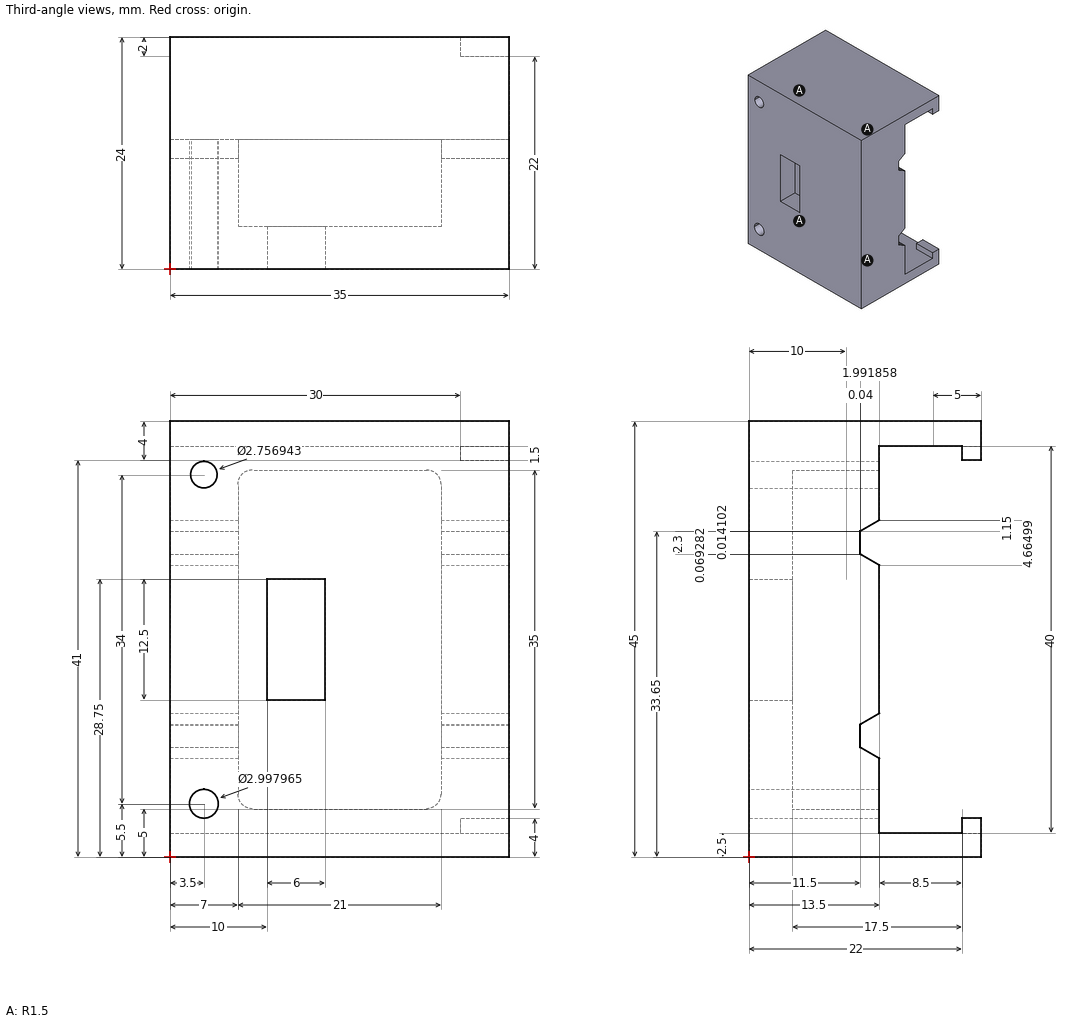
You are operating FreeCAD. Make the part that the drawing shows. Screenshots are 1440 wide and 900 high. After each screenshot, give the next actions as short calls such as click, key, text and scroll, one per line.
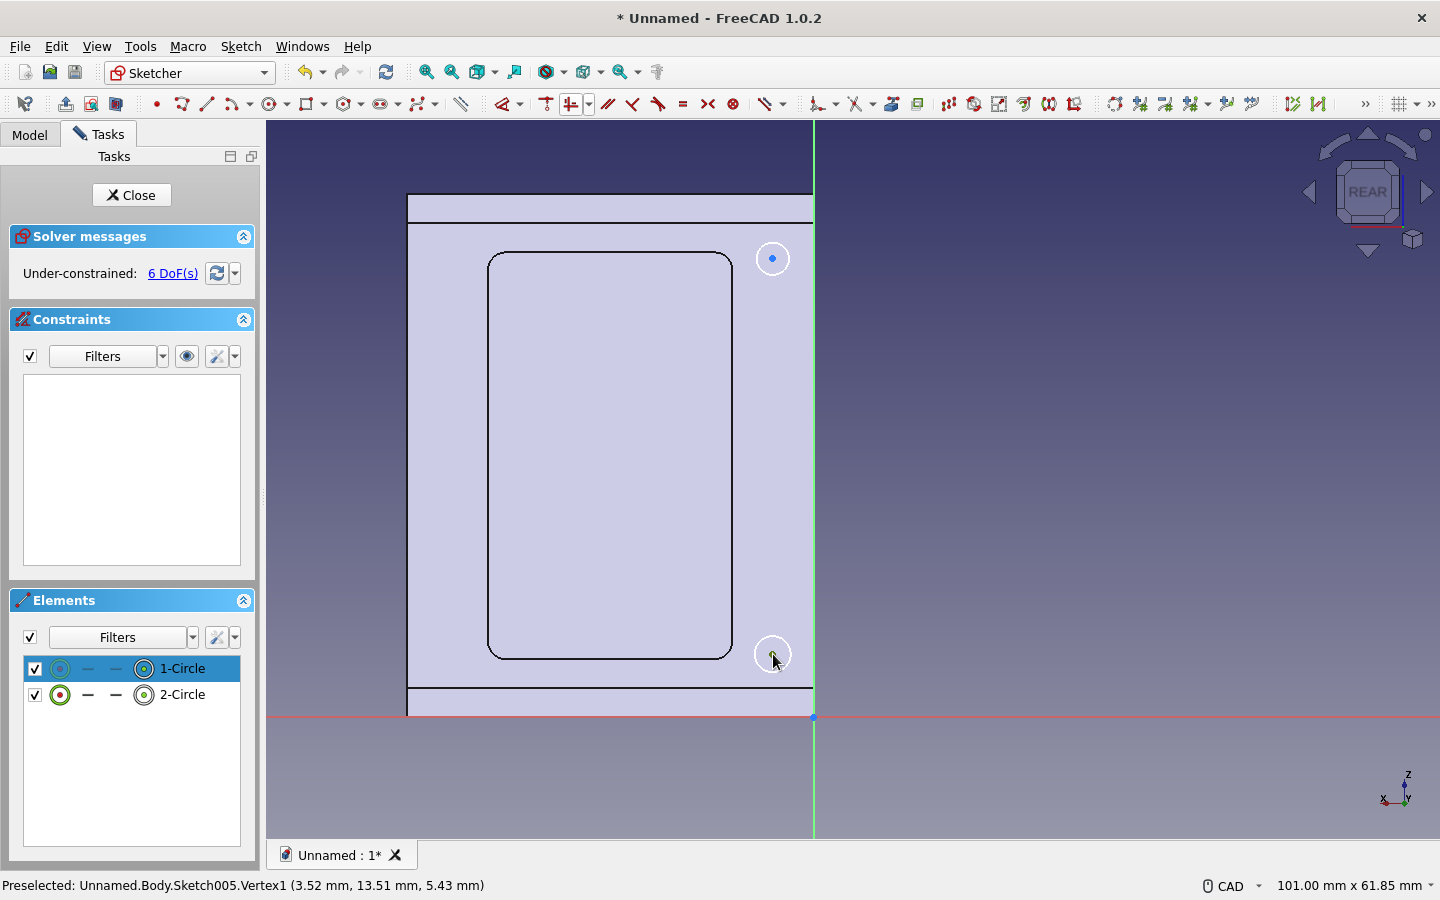
click(773, 259)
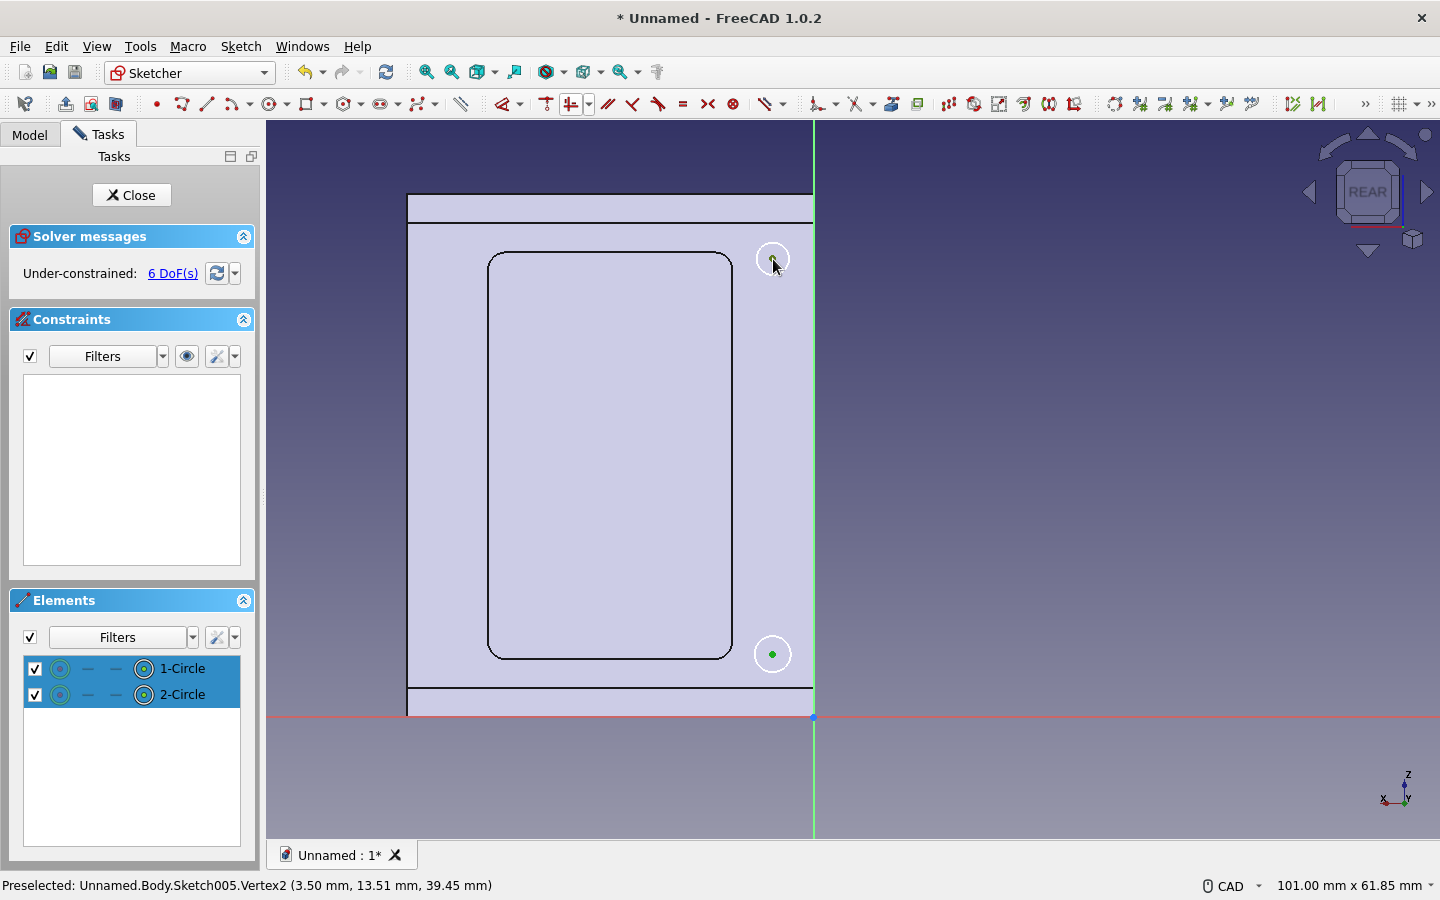
key(v)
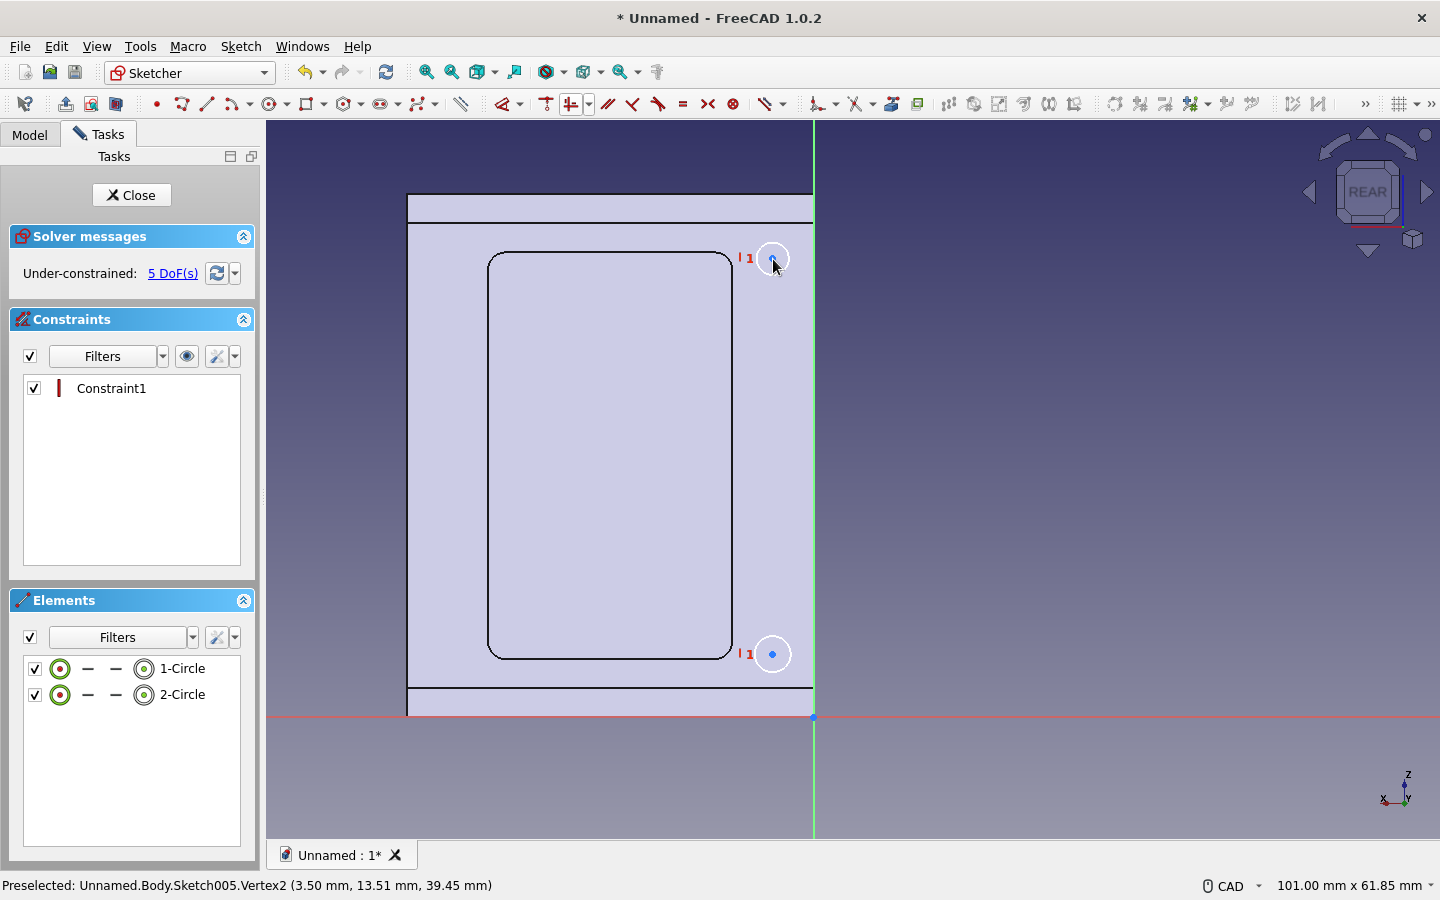
click(502, 104)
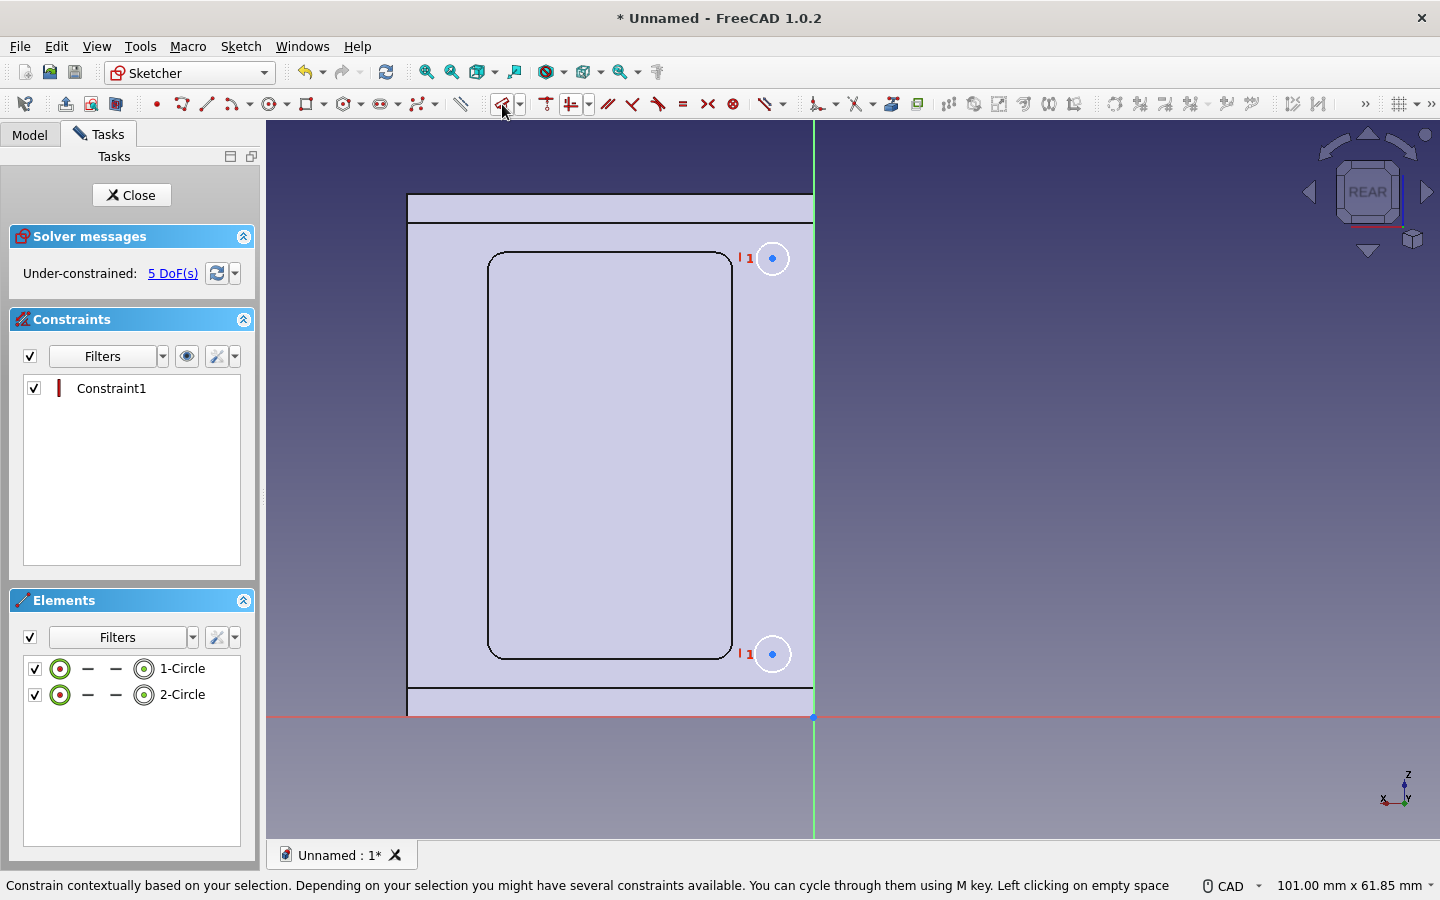
click(785, 641)
click(785, 606)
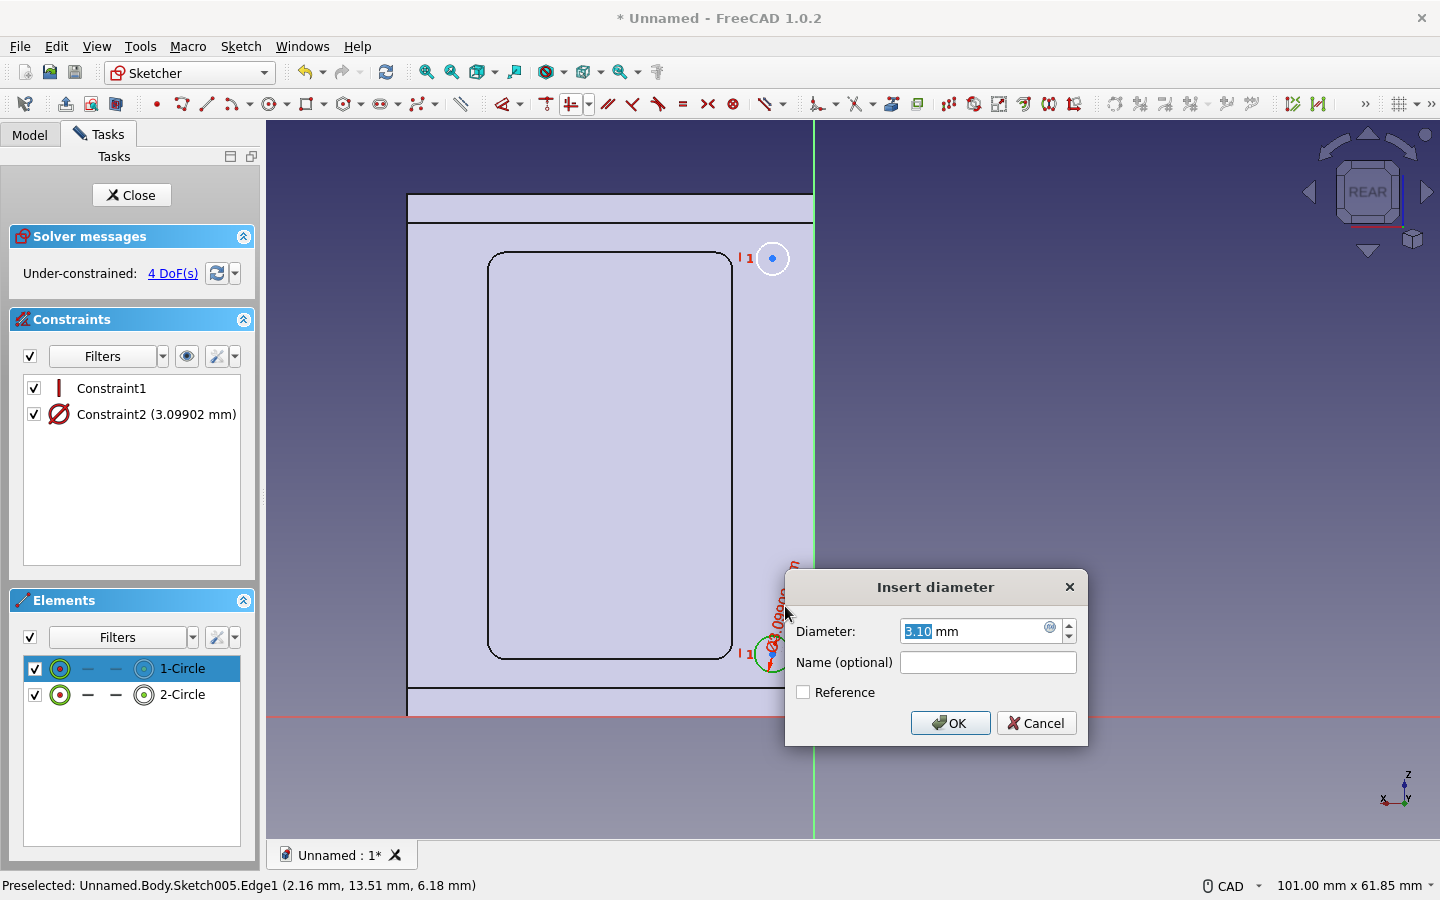
text(2.997965)
key(Return)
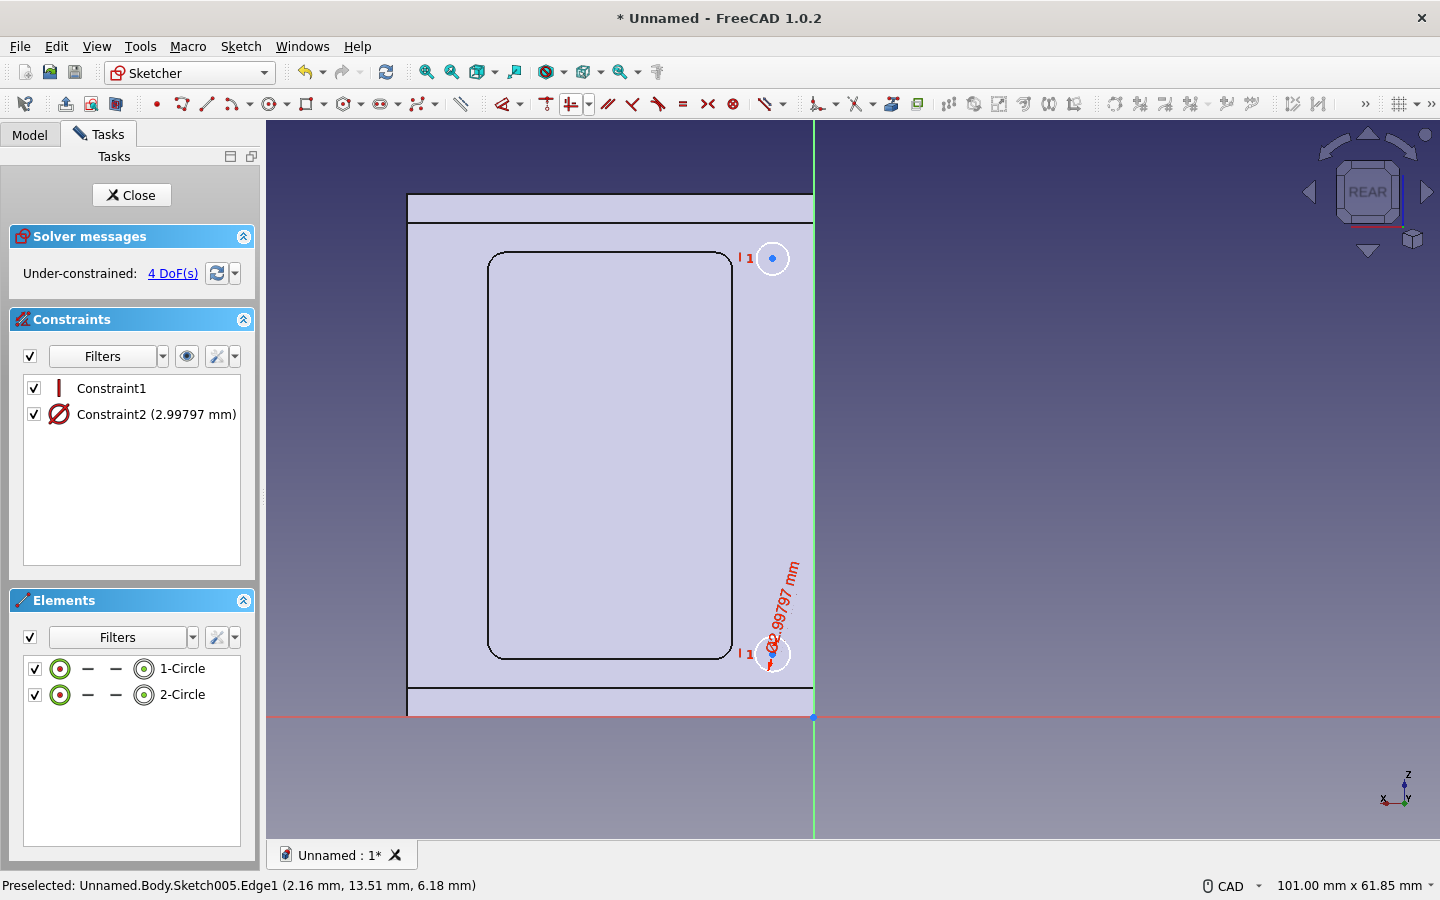
scroll(784, 247, up, 2)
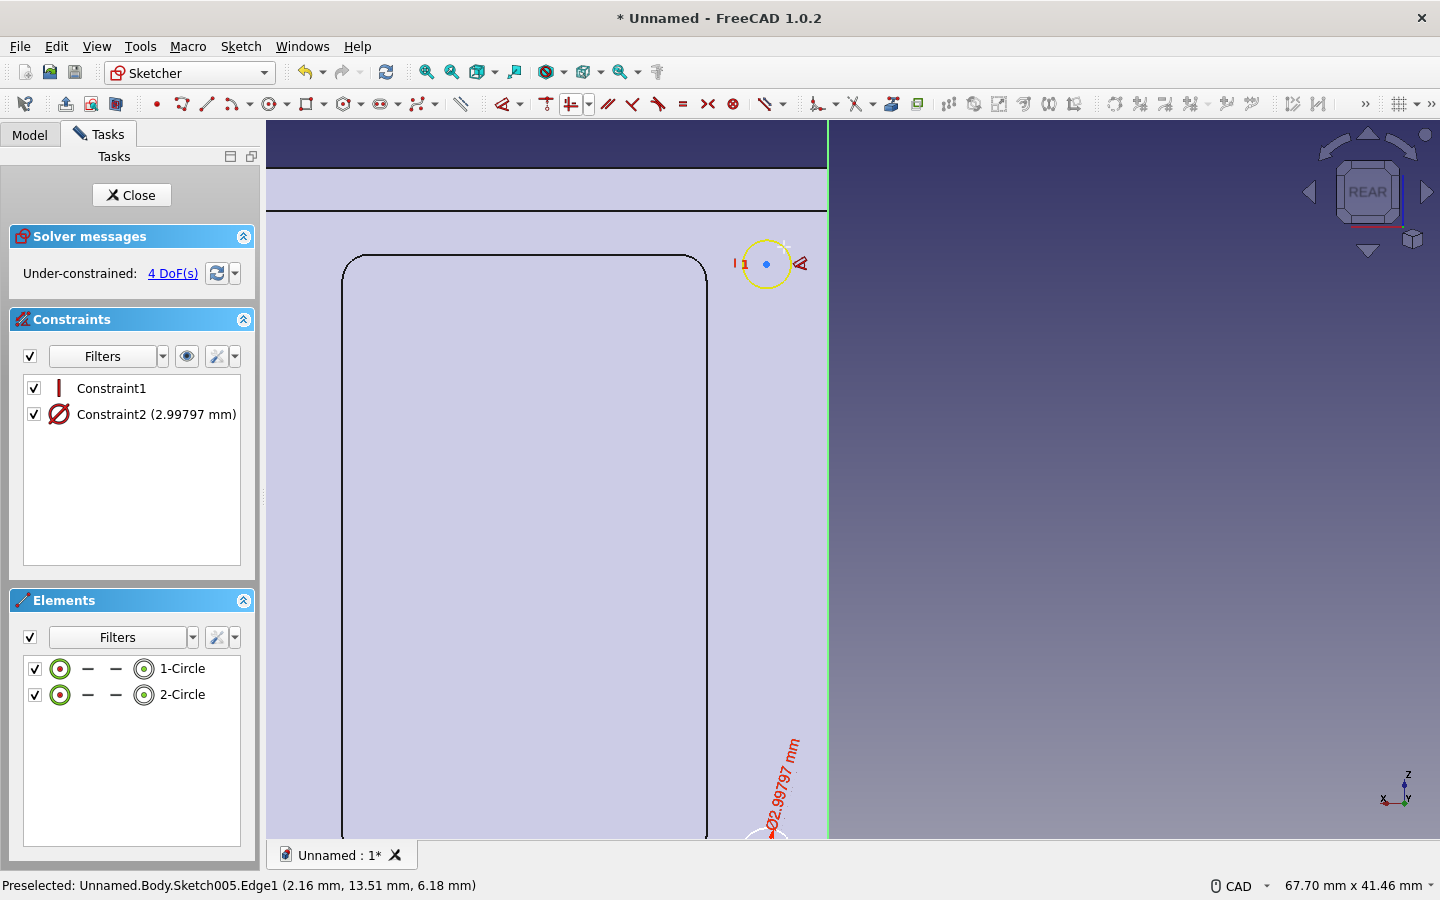
click(784, 247)
click(806, 224)